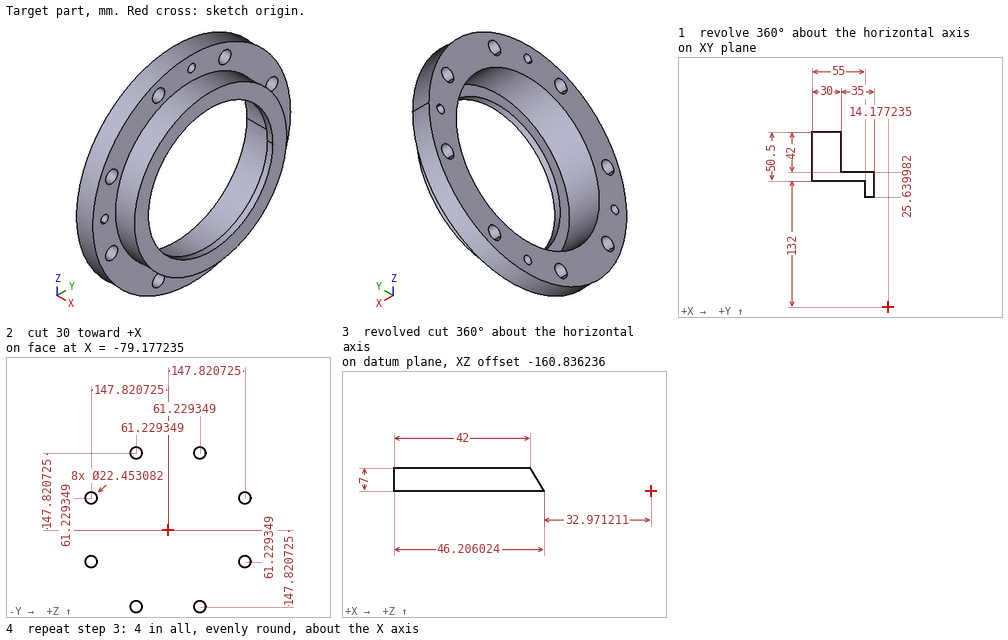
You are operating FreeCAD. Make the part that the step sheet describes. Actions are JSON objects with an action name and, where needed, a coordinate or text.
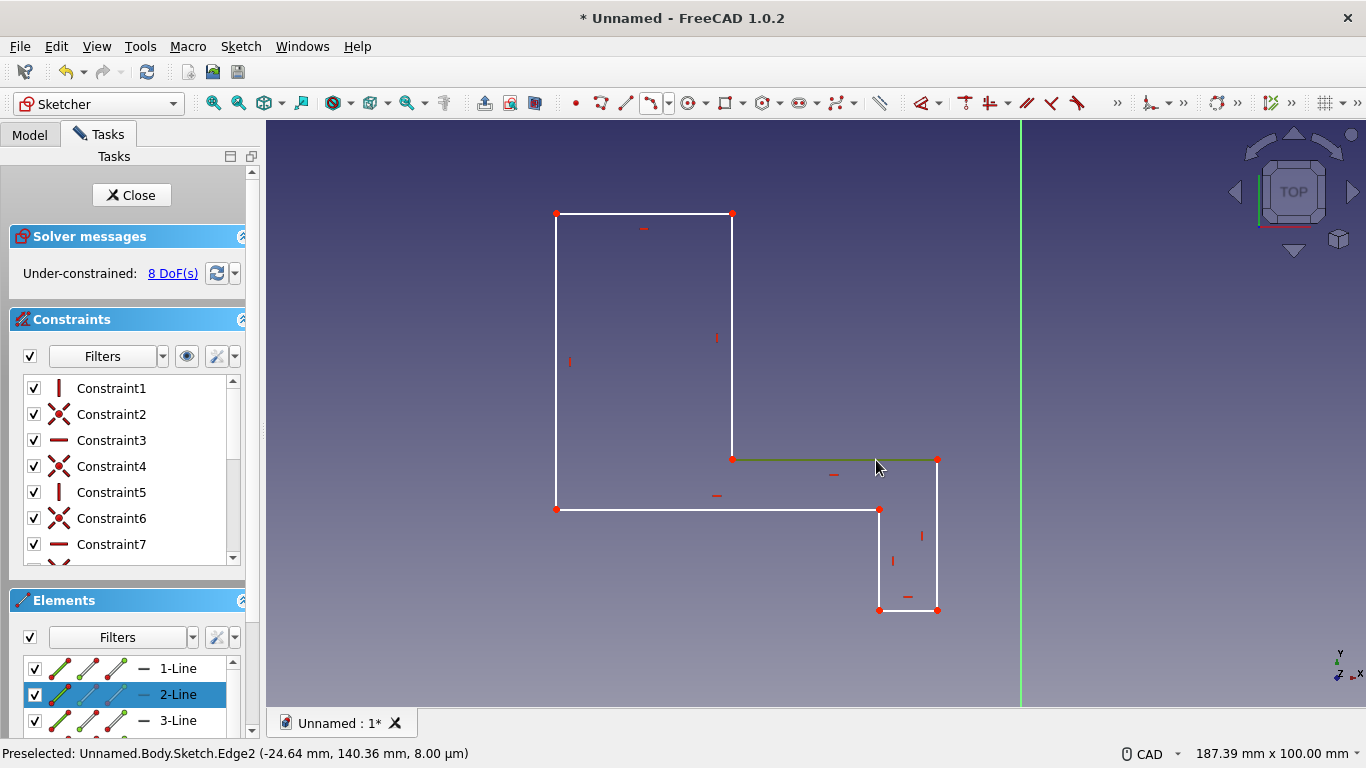
{"action": "key", "text": "l"}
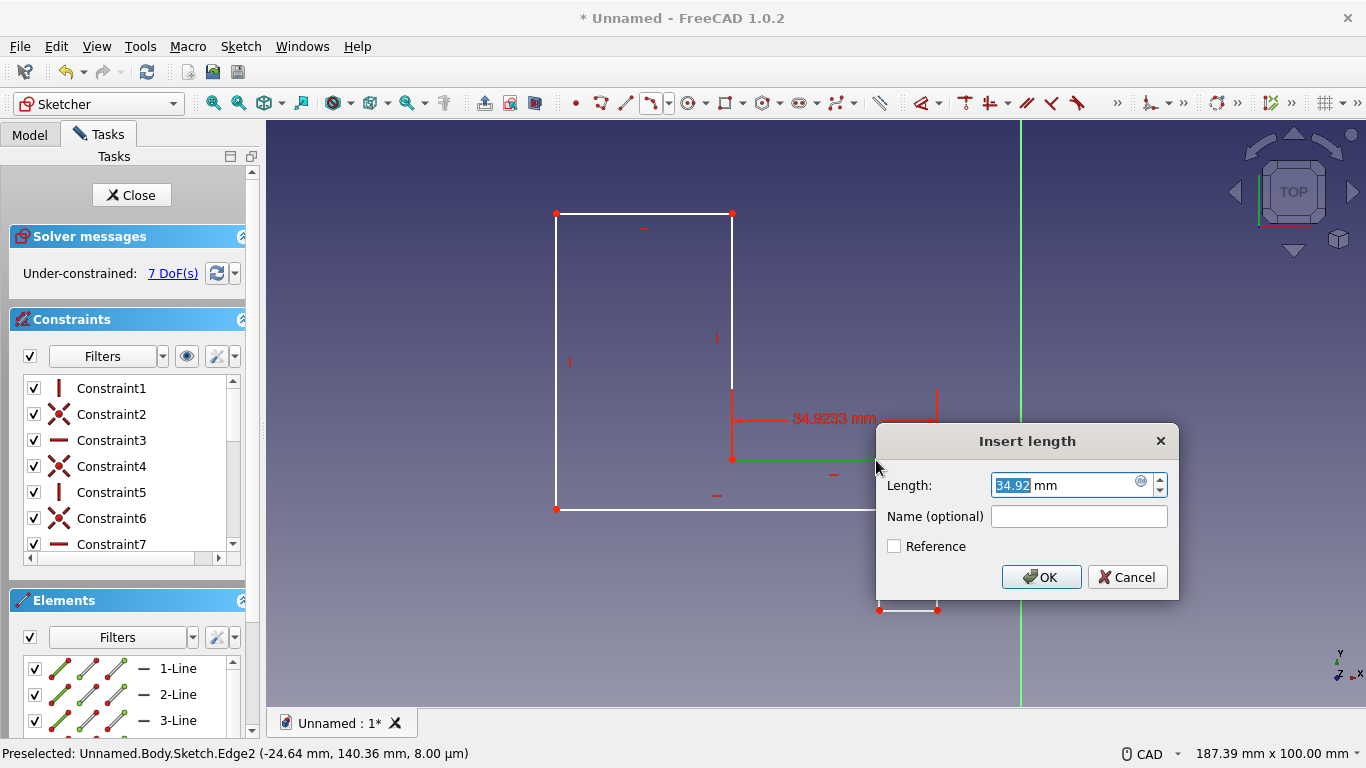
{"action": "type", "text": "35"}
{"action": "key", "text": "Return"}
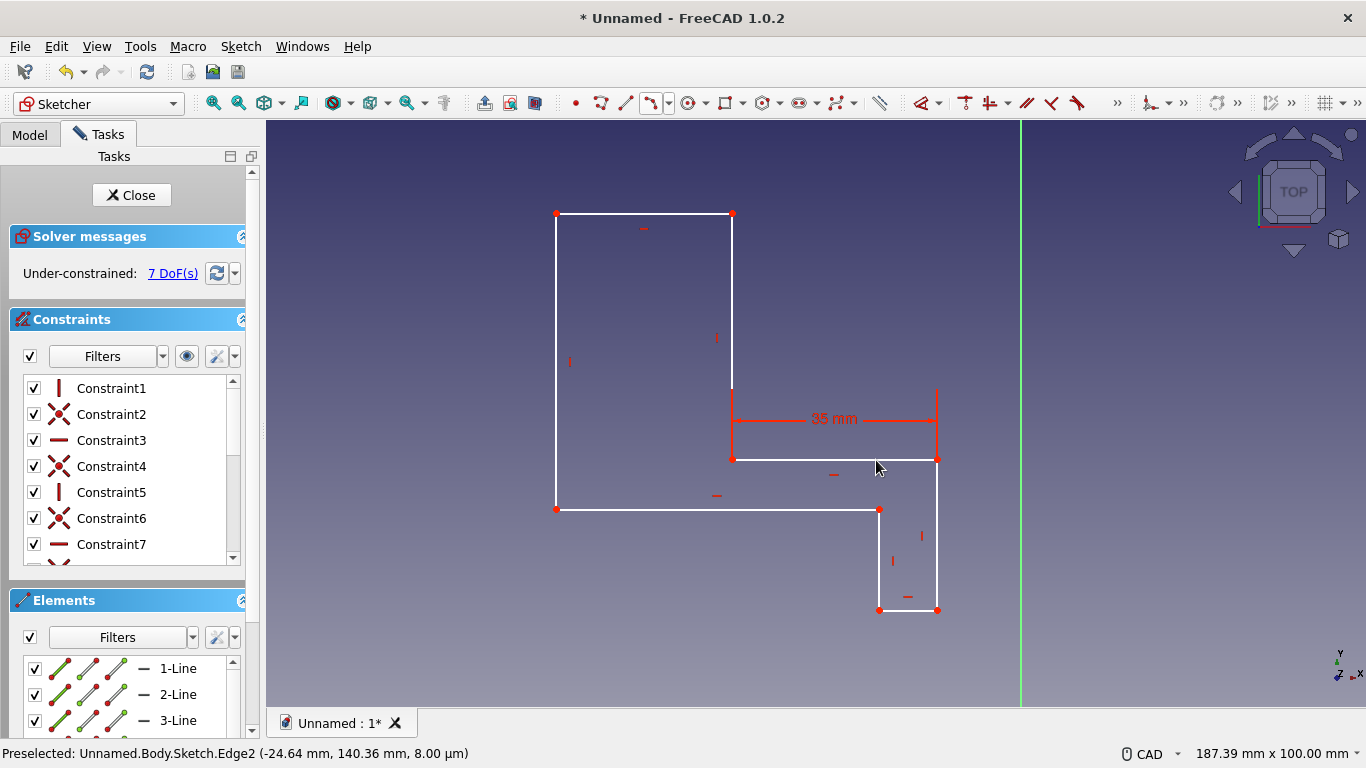
{"action": "left_click", "coordinate": [732, 386]}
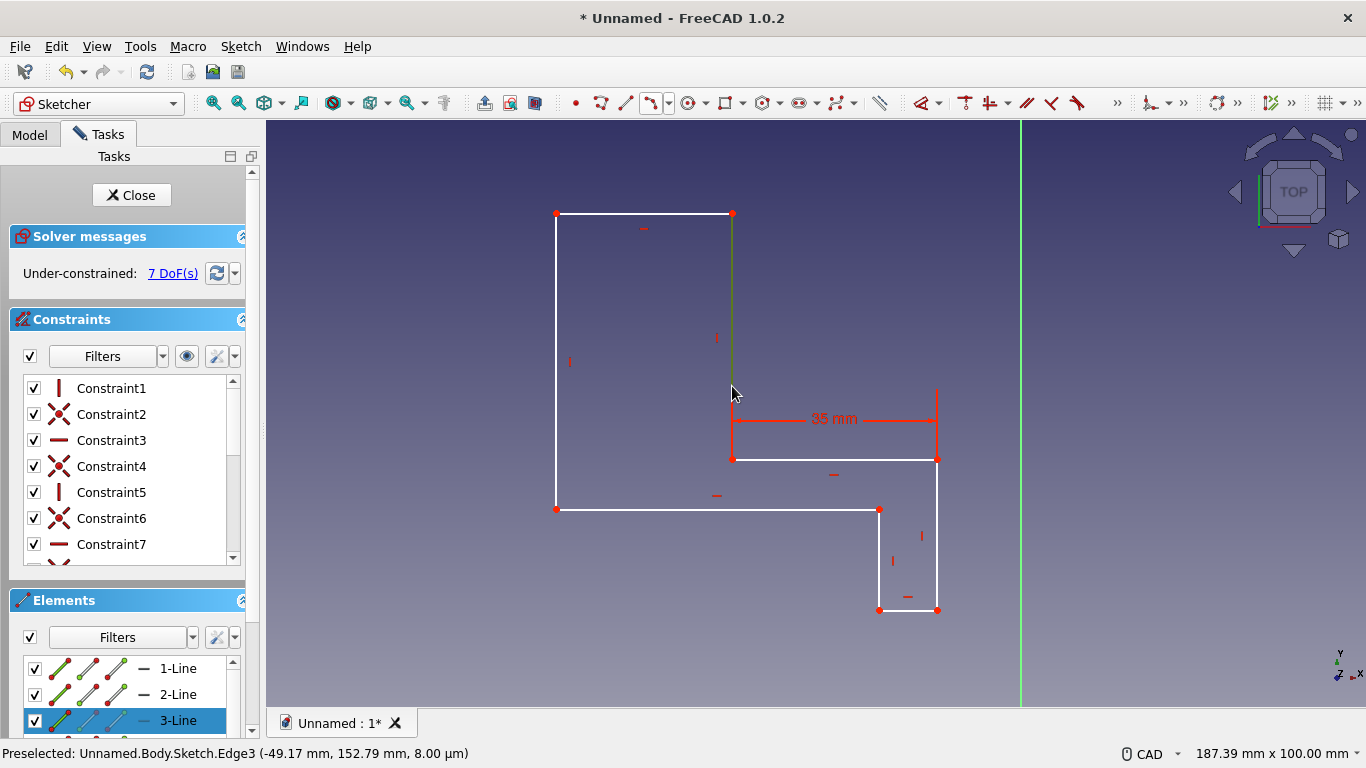
{"action": "left_click", "coordinate": [938, 104]}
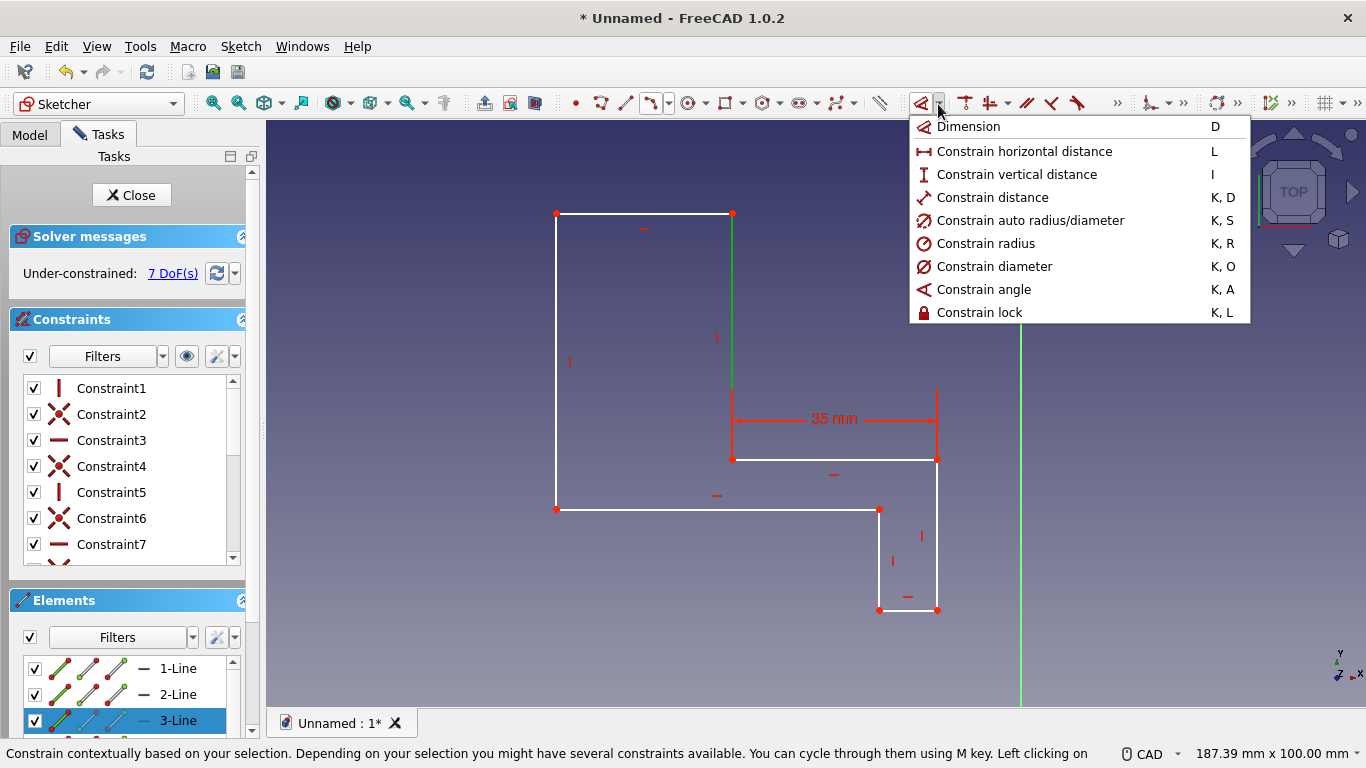
{"action": "left_click", "coordinate": [1080, 174]}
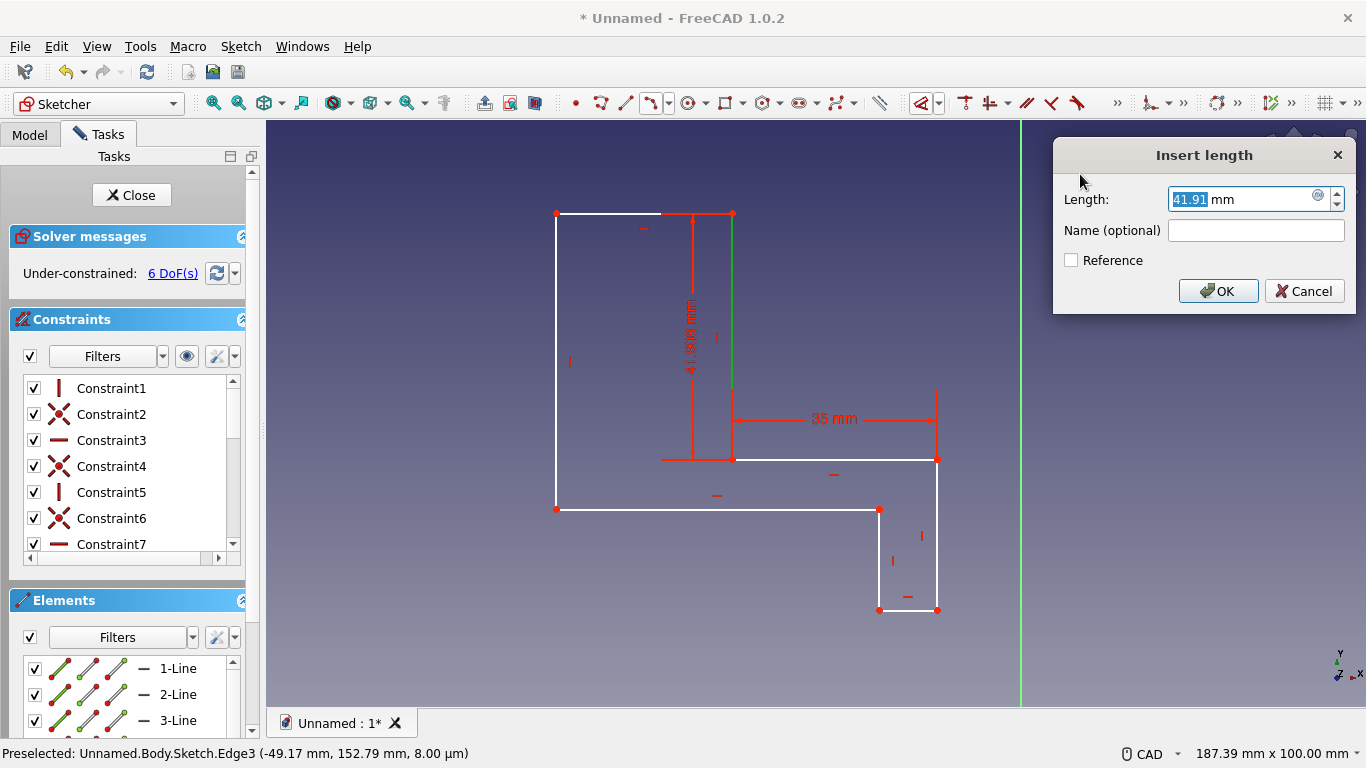
{"action": "type", "text": "42"}
{"action": "key", "text": "Return"}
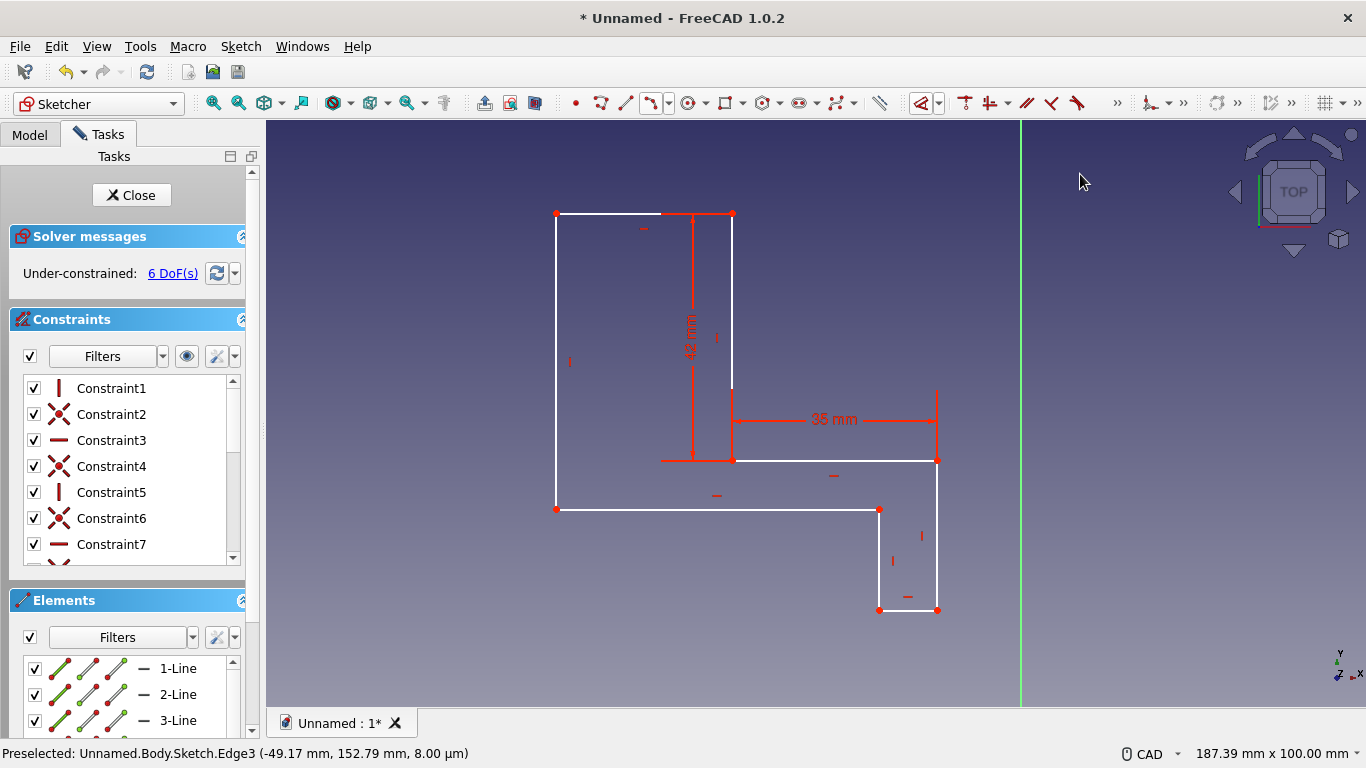
{"action": "left_click", "coordinate": [679, 214]}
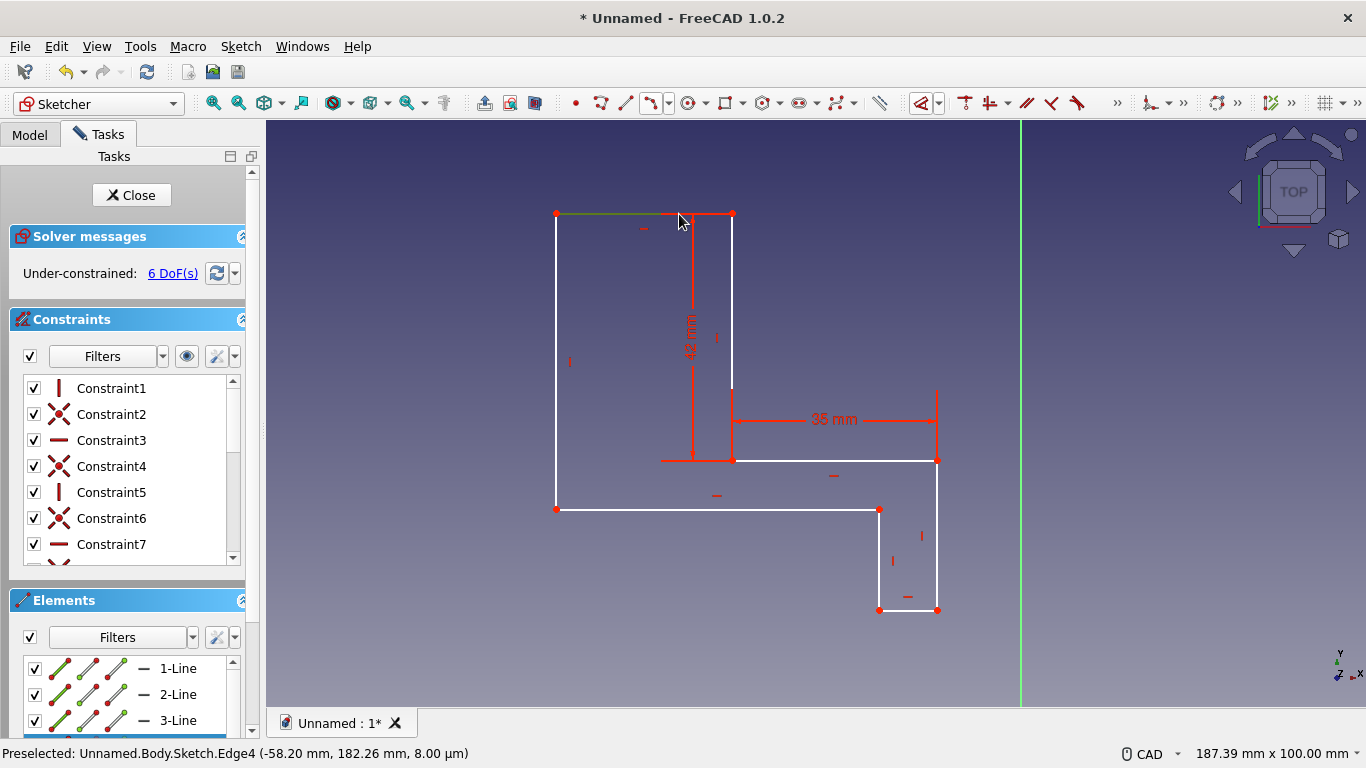
{"action": "key", "text": "l"}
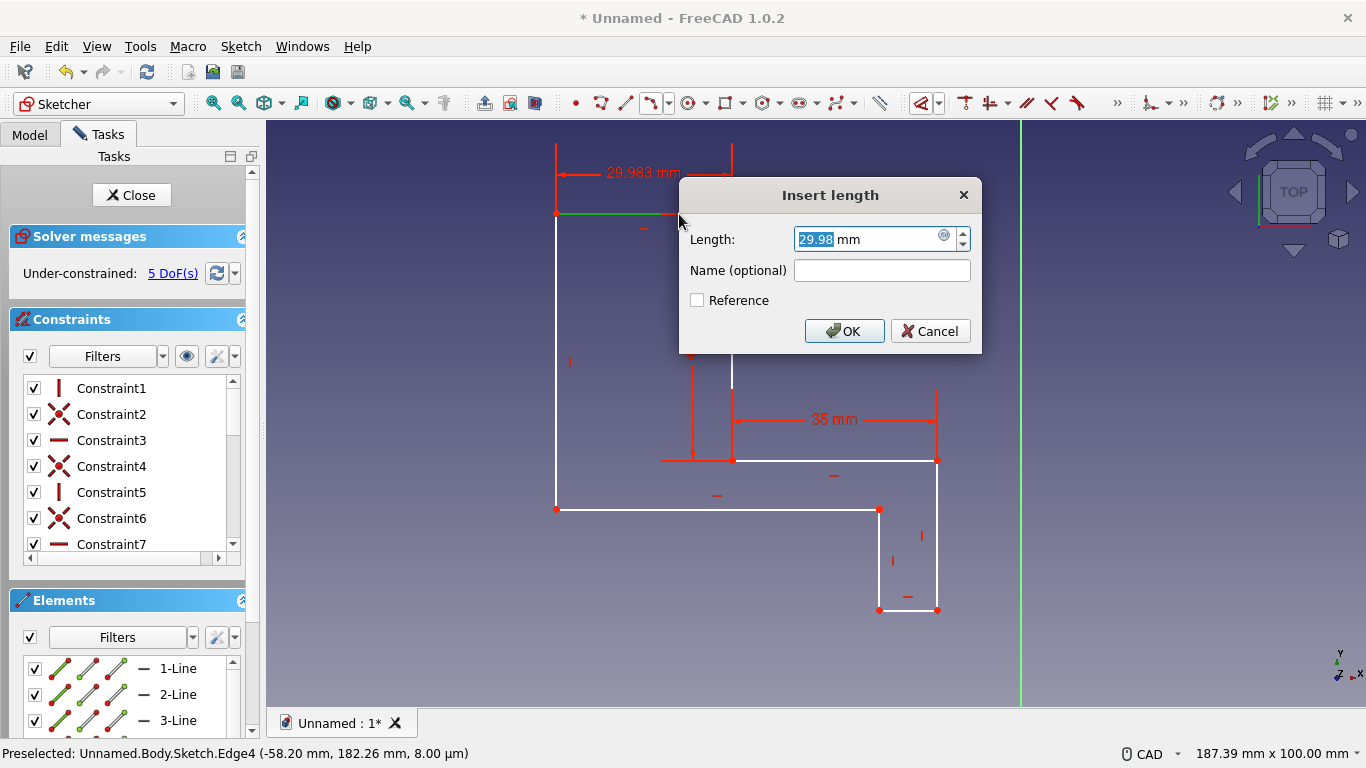
{"action": "type", "text": "30"}
{"action": "key", "text": "Return"}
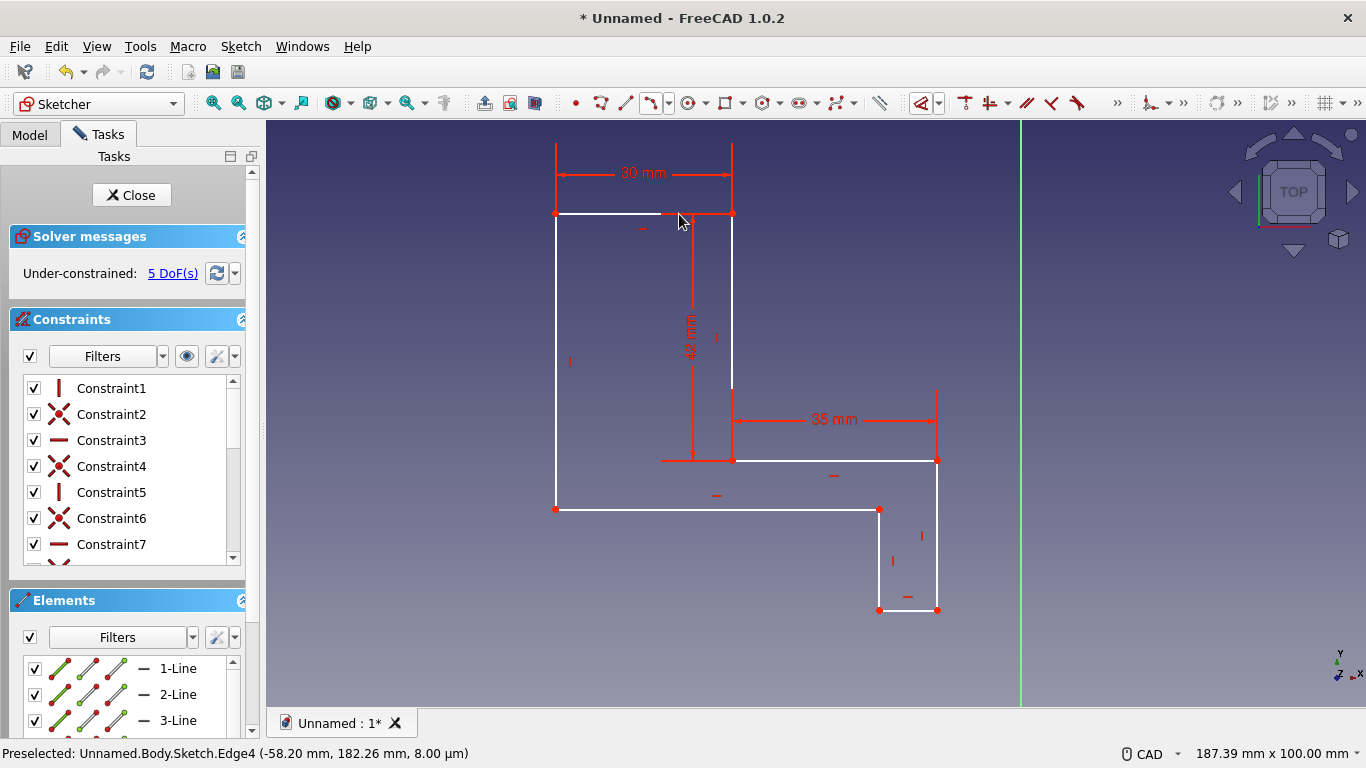
{"action": "left_click", "coordinate": [653, 510]}